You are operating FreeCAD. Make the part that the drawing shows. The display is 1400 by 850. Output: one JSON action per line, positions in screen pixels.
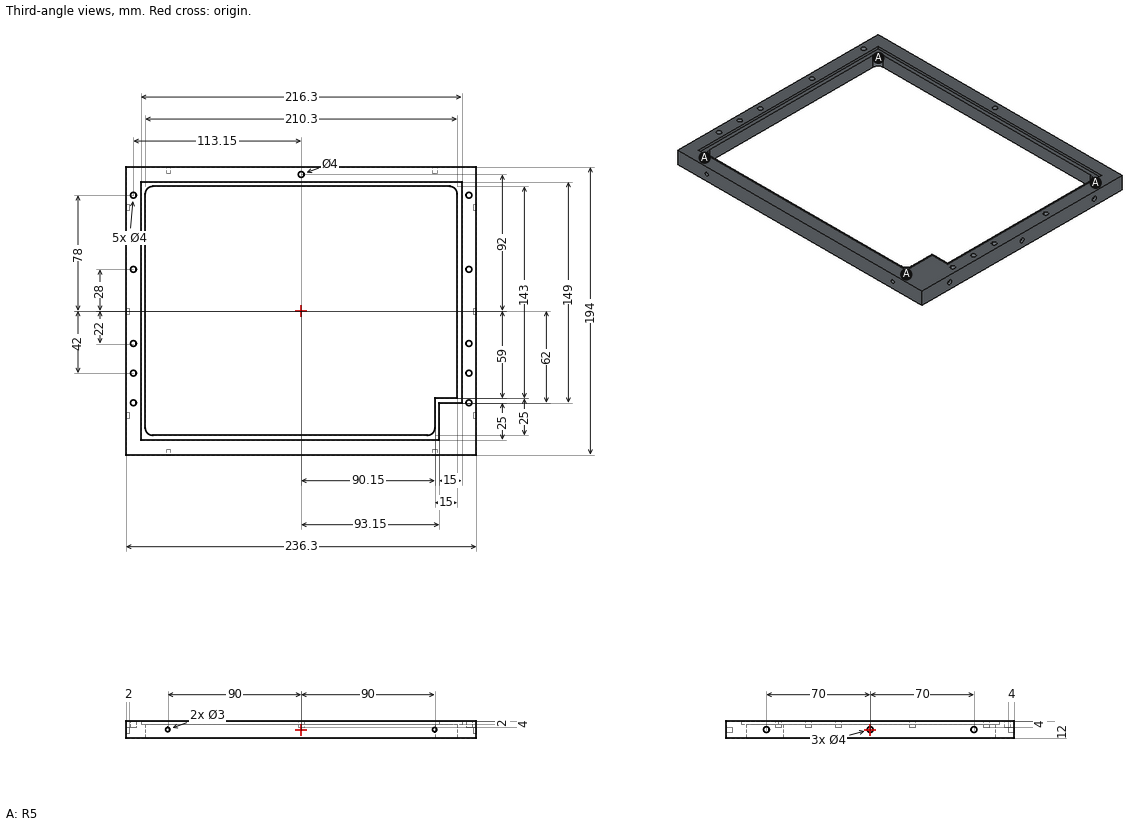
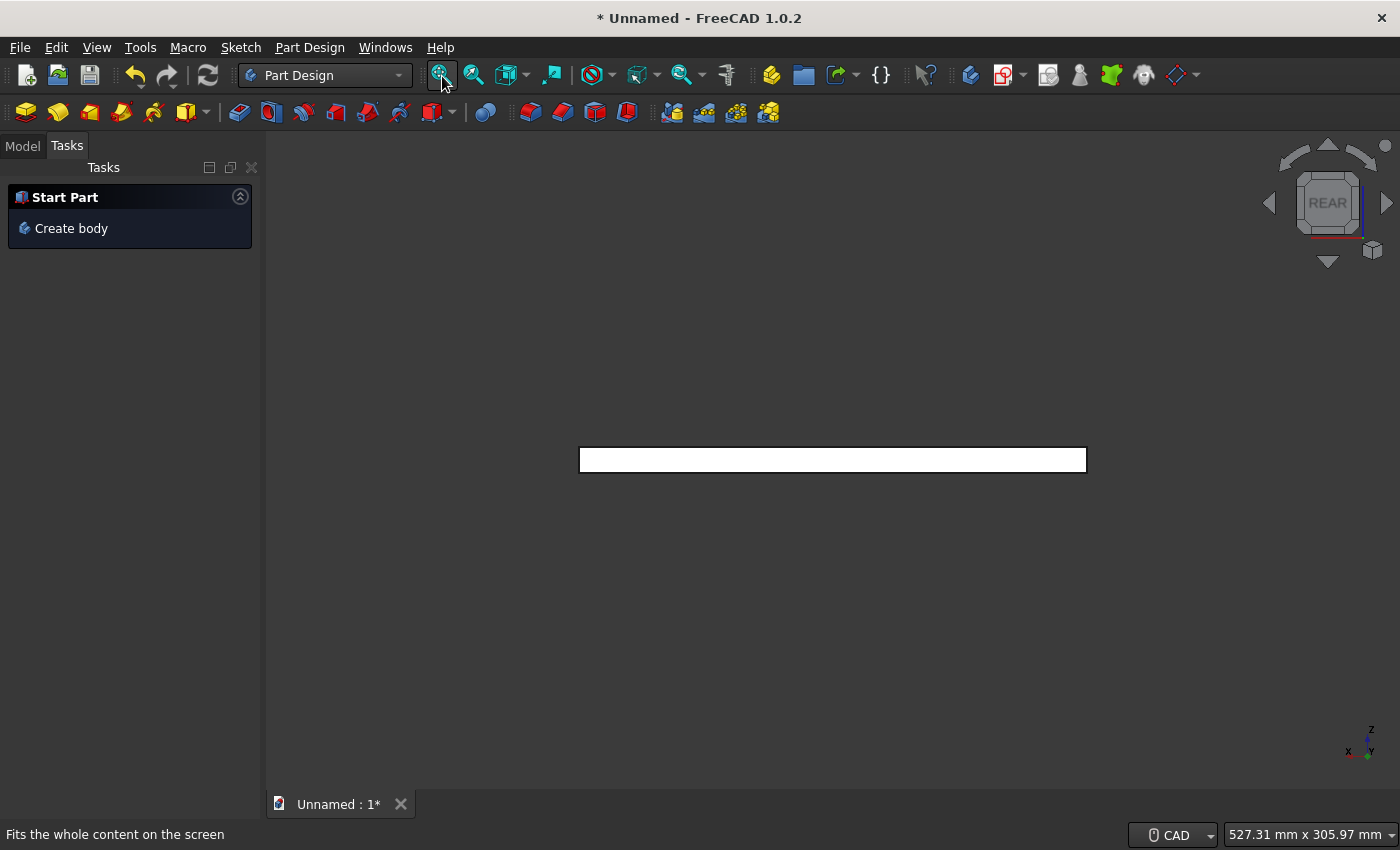
{"action": "key", "text": "6"}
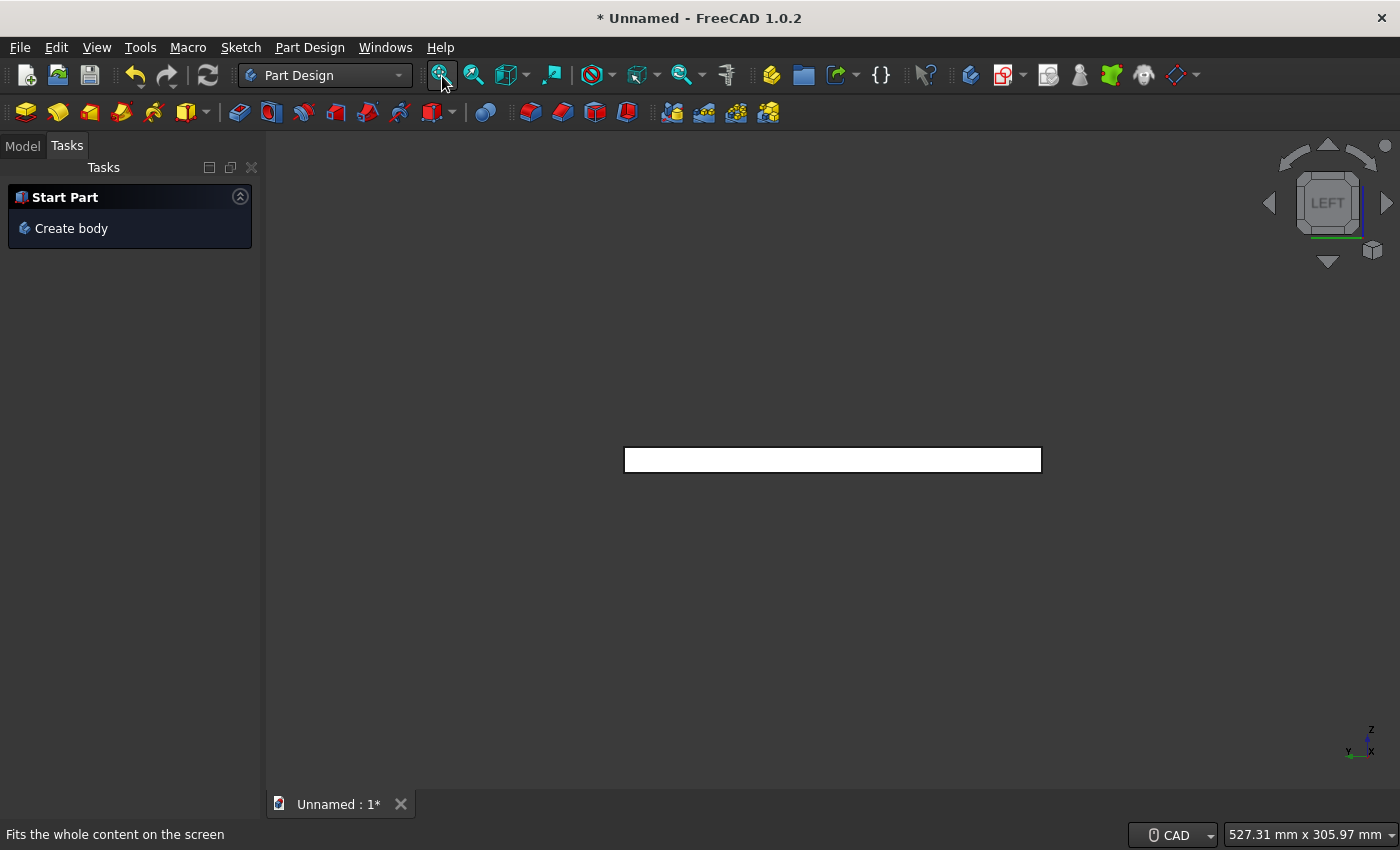
{"action": "left_click", "coordinate": [442, 76]}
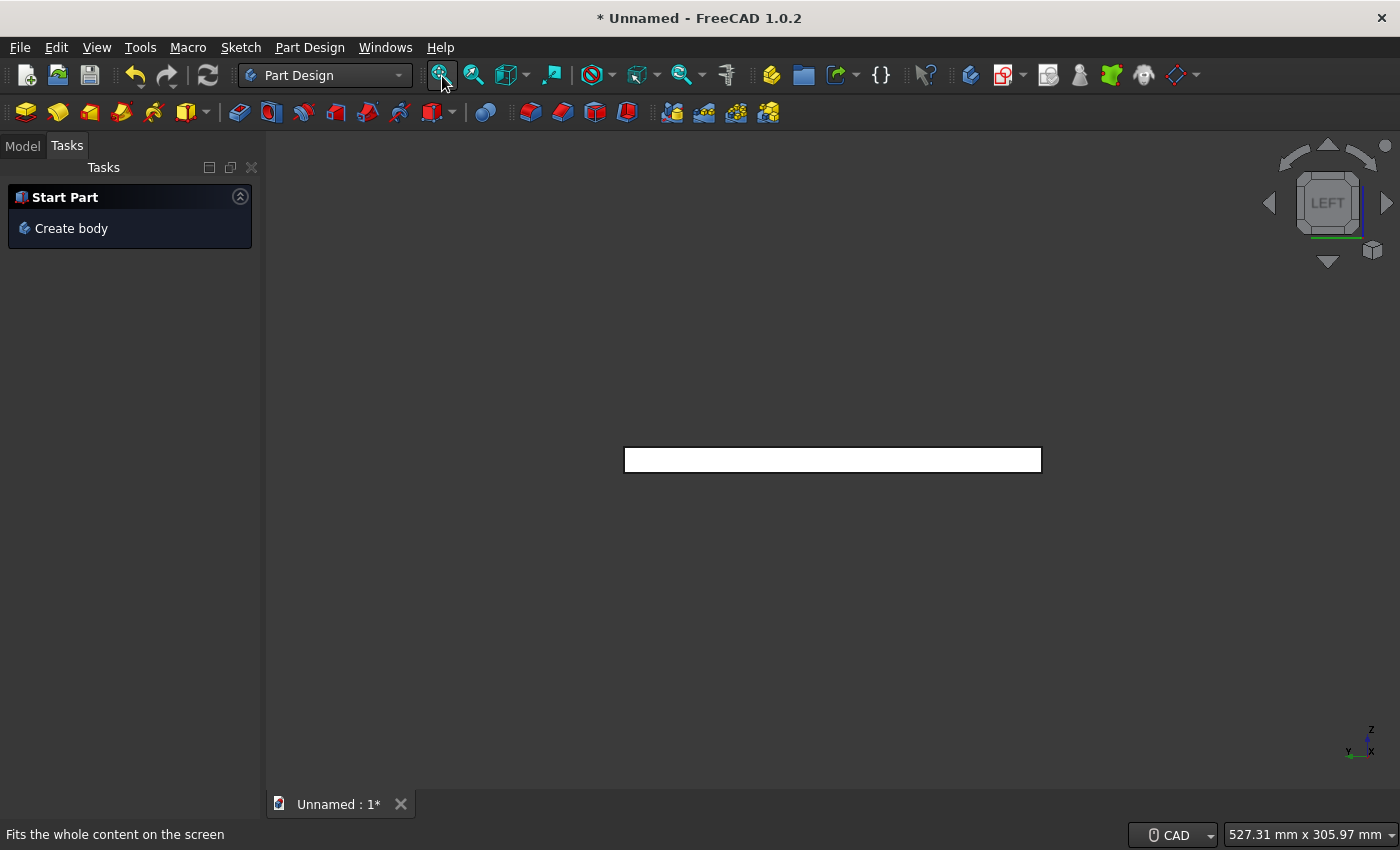
{"action": "scroll", "coordinate": [1014, 461], "scroll_direction": "up", "scroll_amount": 4}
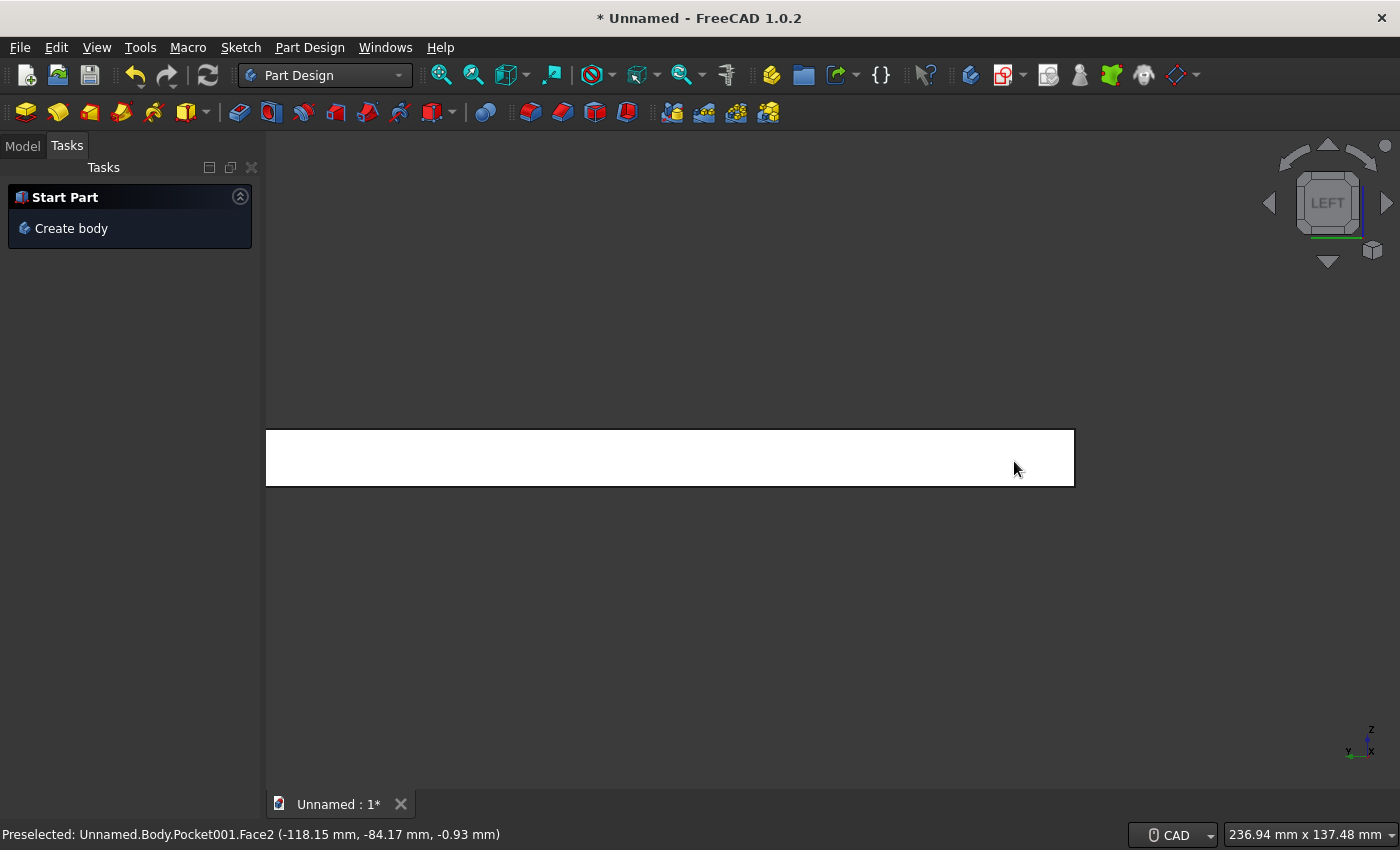
{"action": "left_click", "coordinate": [442, 76]}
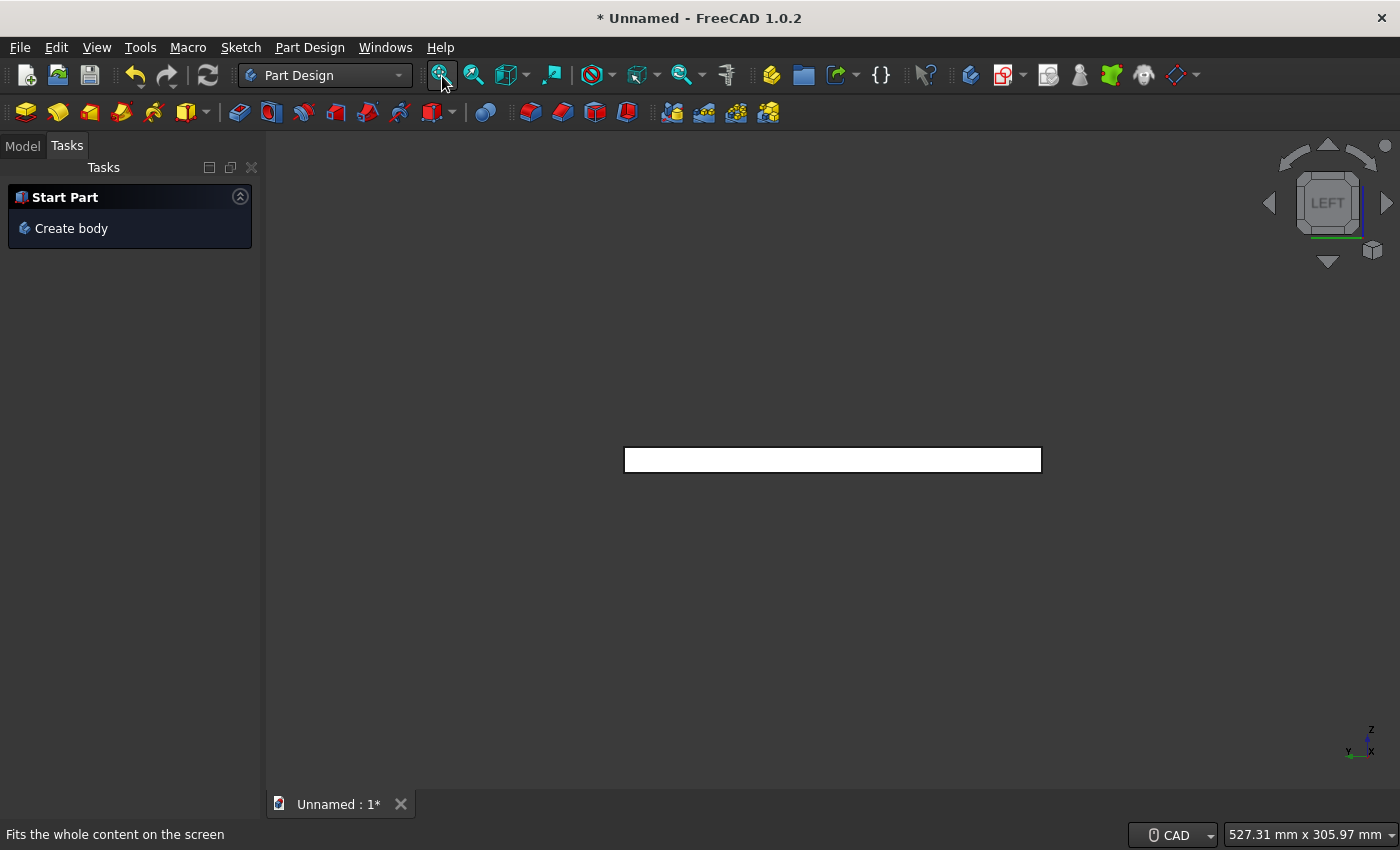
{"action": "key", "text": "v 3"}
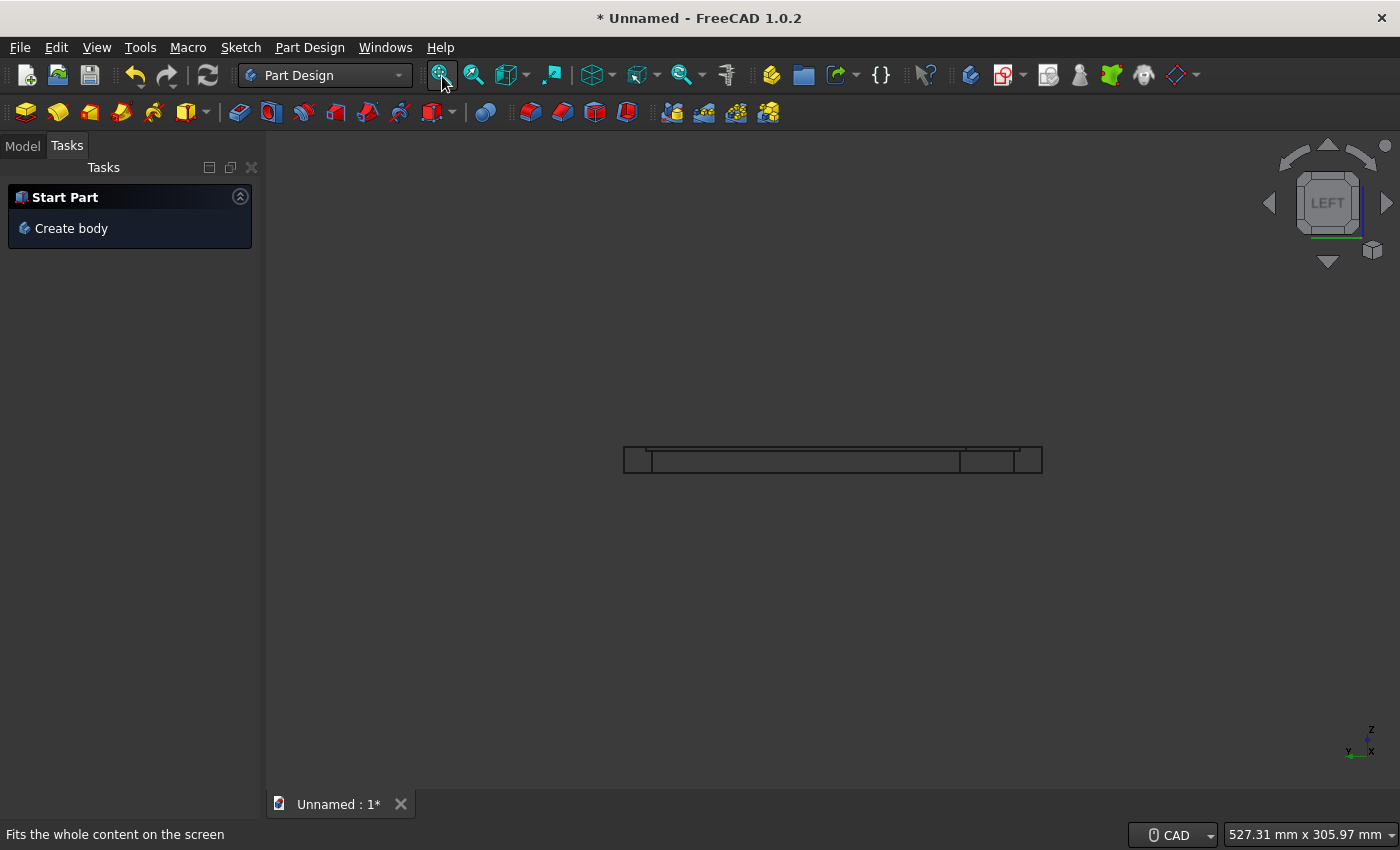
{"action": "key", "text": "0"}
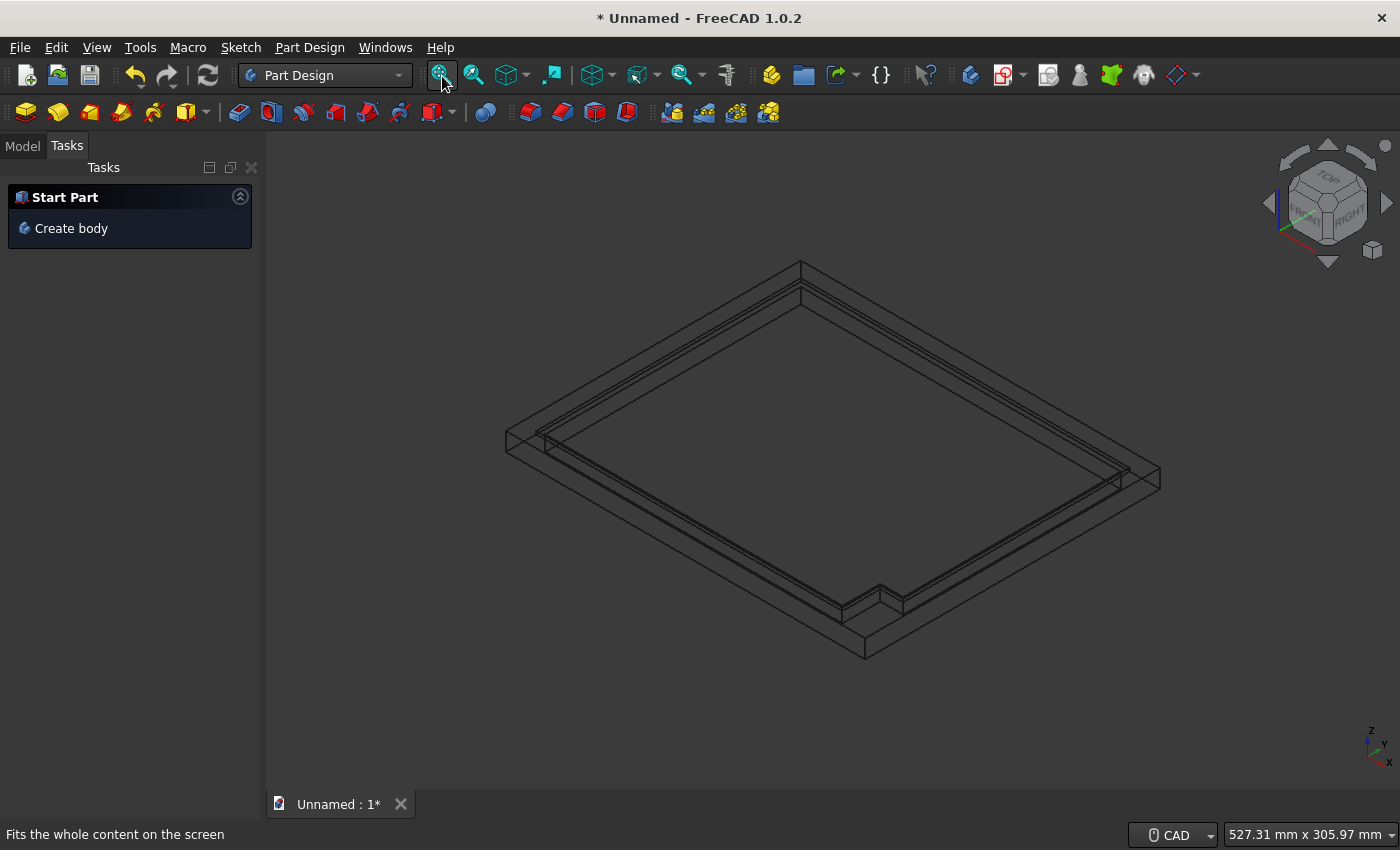
{"action": "left_click", "coordinate": [801, 295]}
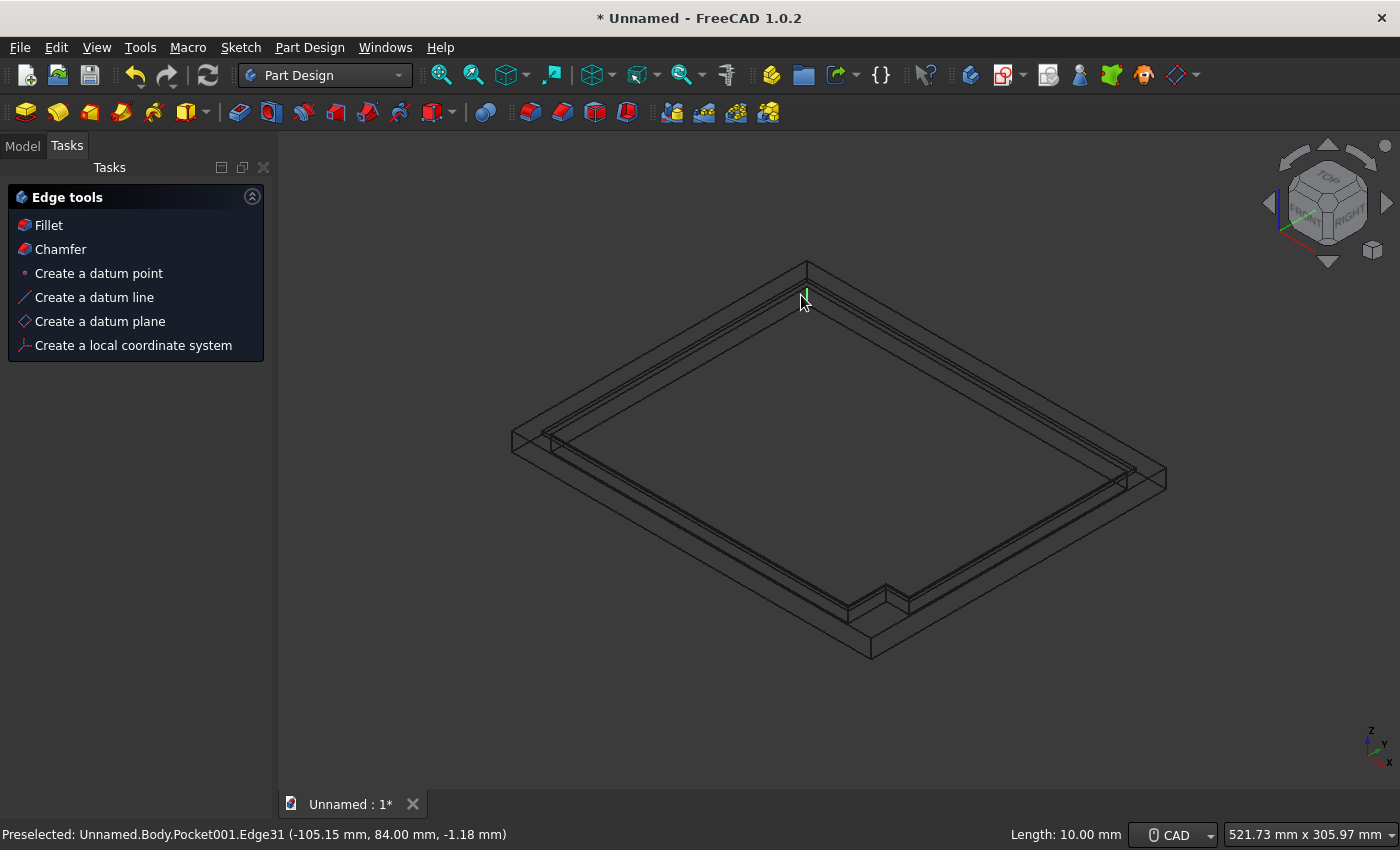
{"action": "scroll", "coordinate": [848, 614], "scroll_direction": "up", "scroll_amount": 4}